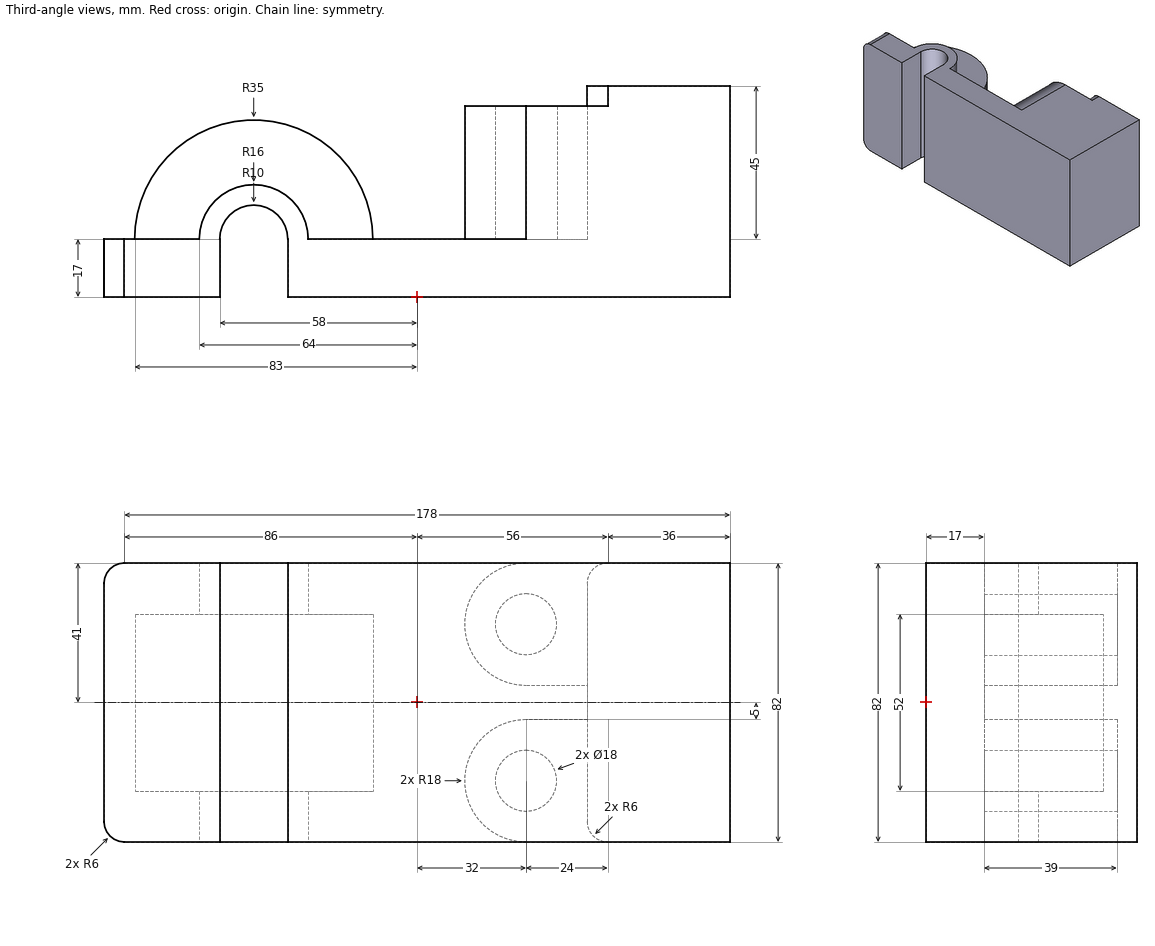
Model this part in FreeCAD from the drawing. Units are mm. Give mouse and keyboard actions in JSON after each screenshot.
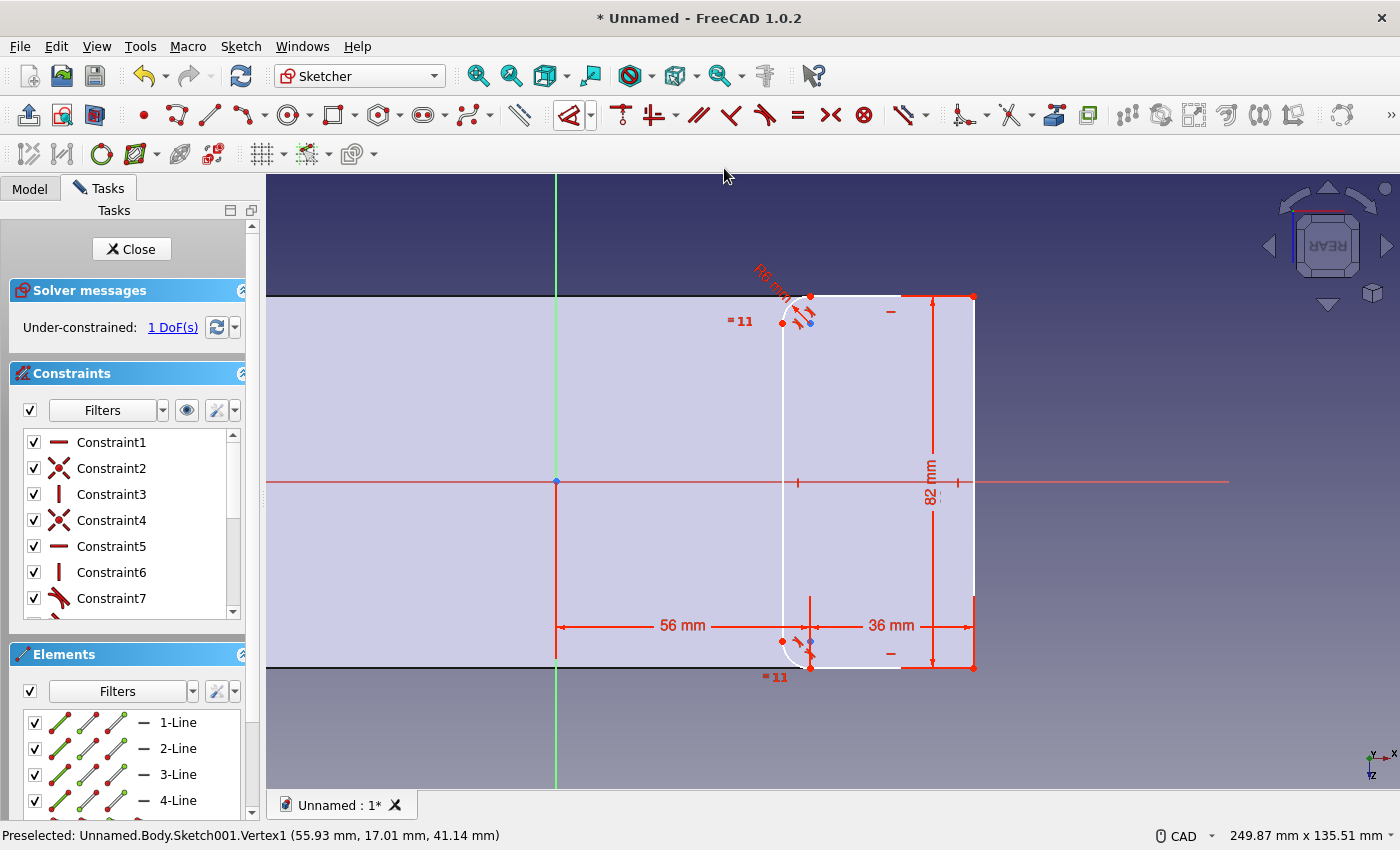
{"action": "left_click", "coordinate": [810, 668]}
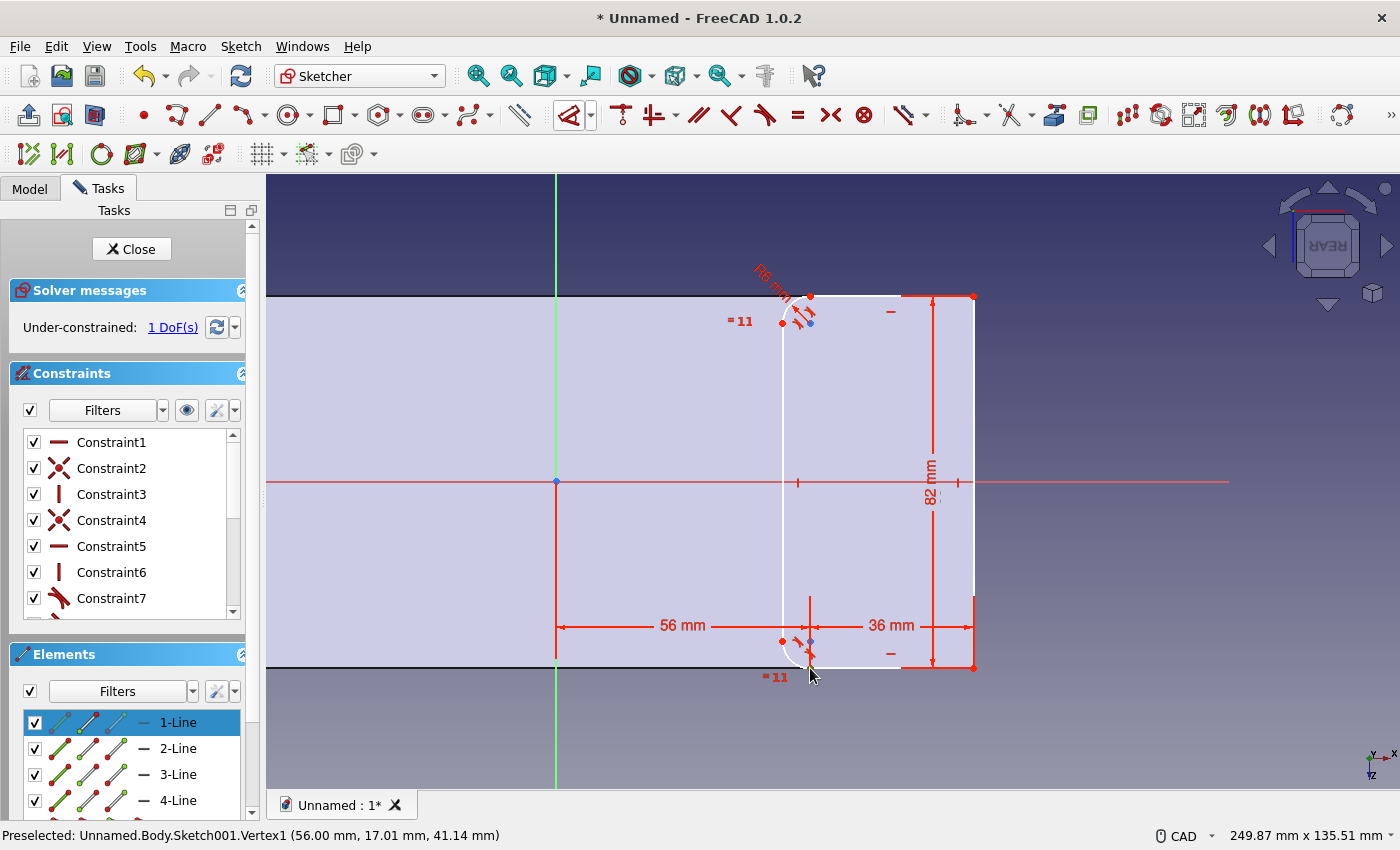
{"action": "key", "text": "i"}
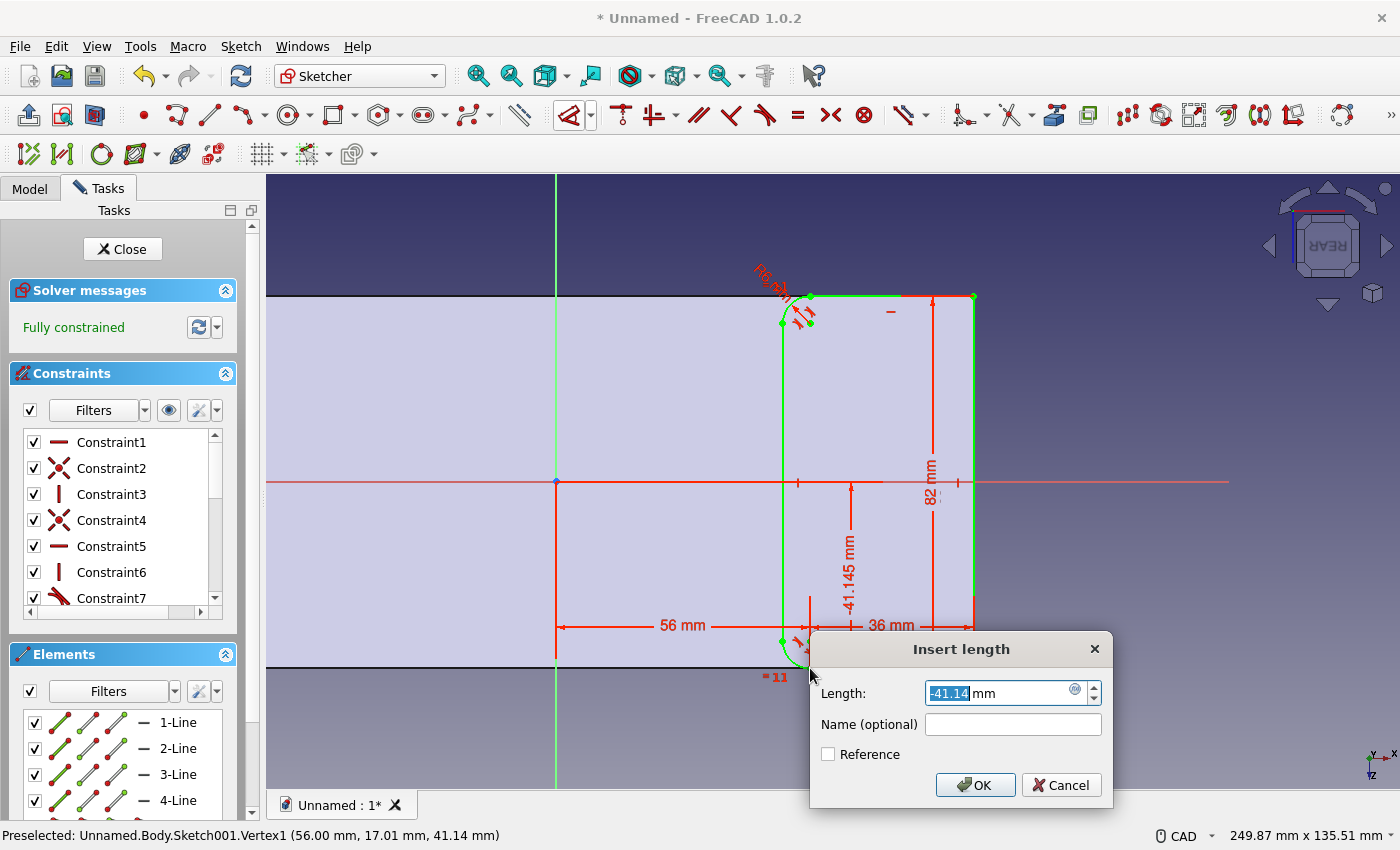
{"action": "type", "text": "-41"}
{"action": "key", "text": "Return"}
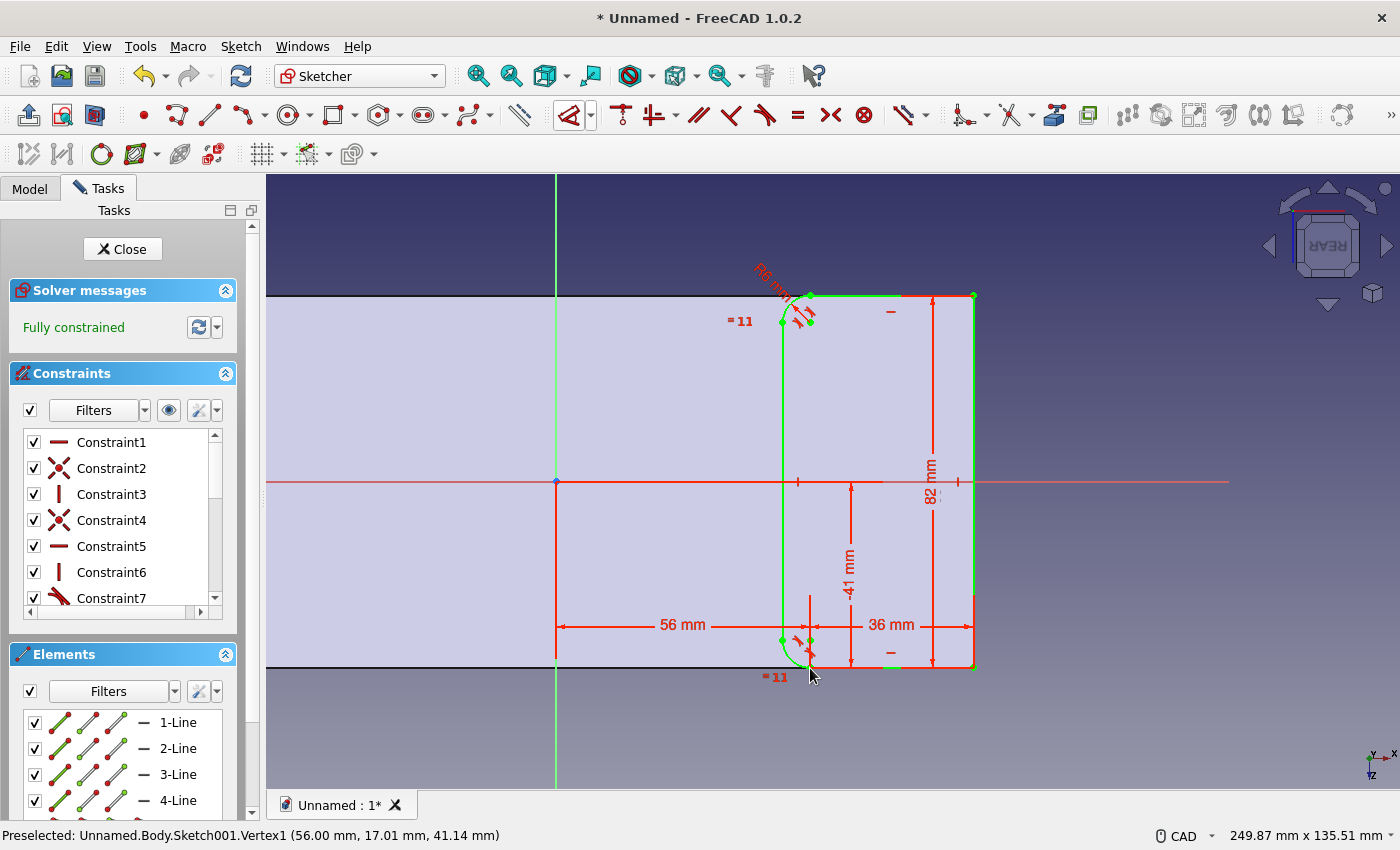
{"action": "left_click", "coordinate": [123, 249]}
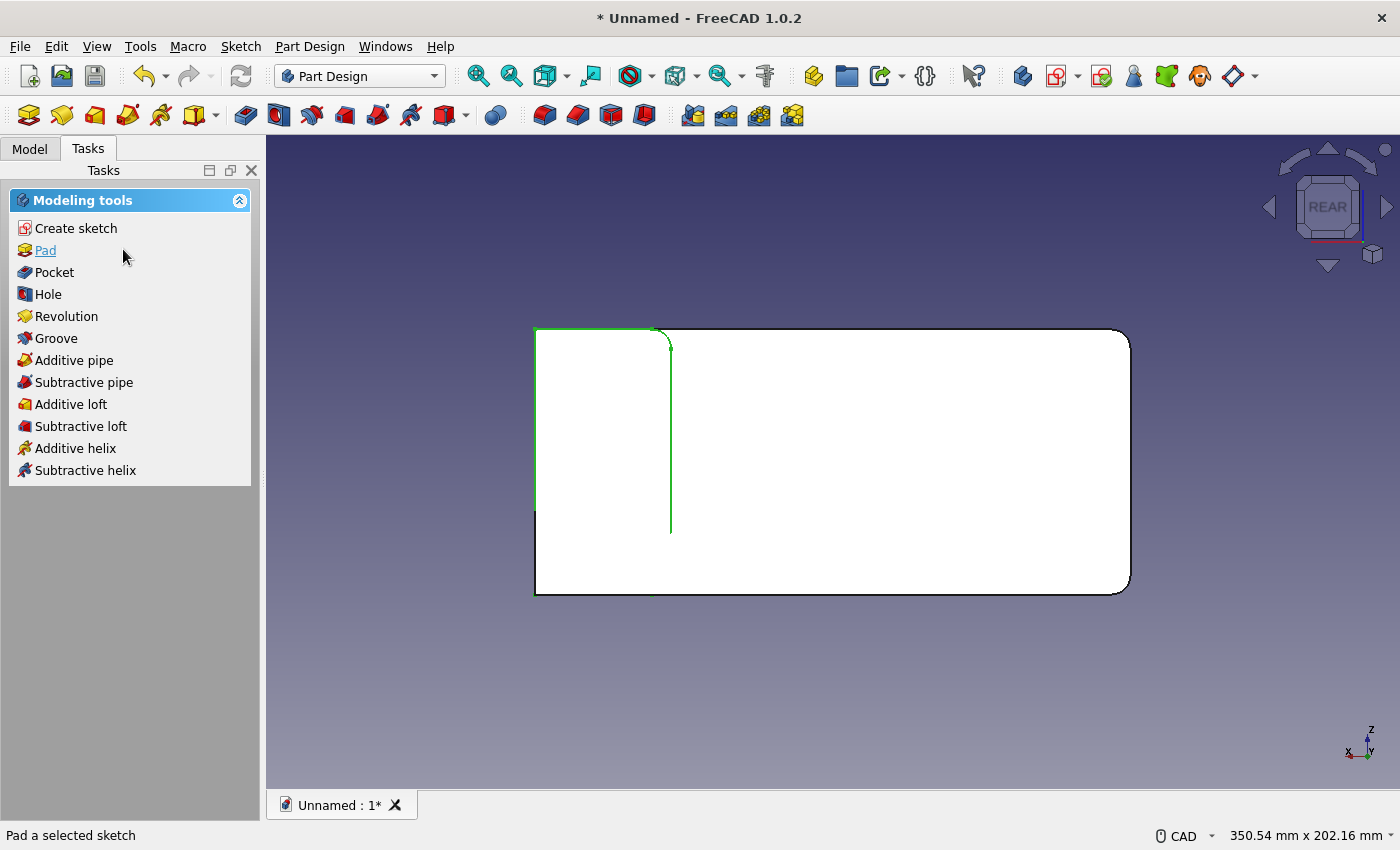
{"action": "left_click", "coordinate": [29, 116]}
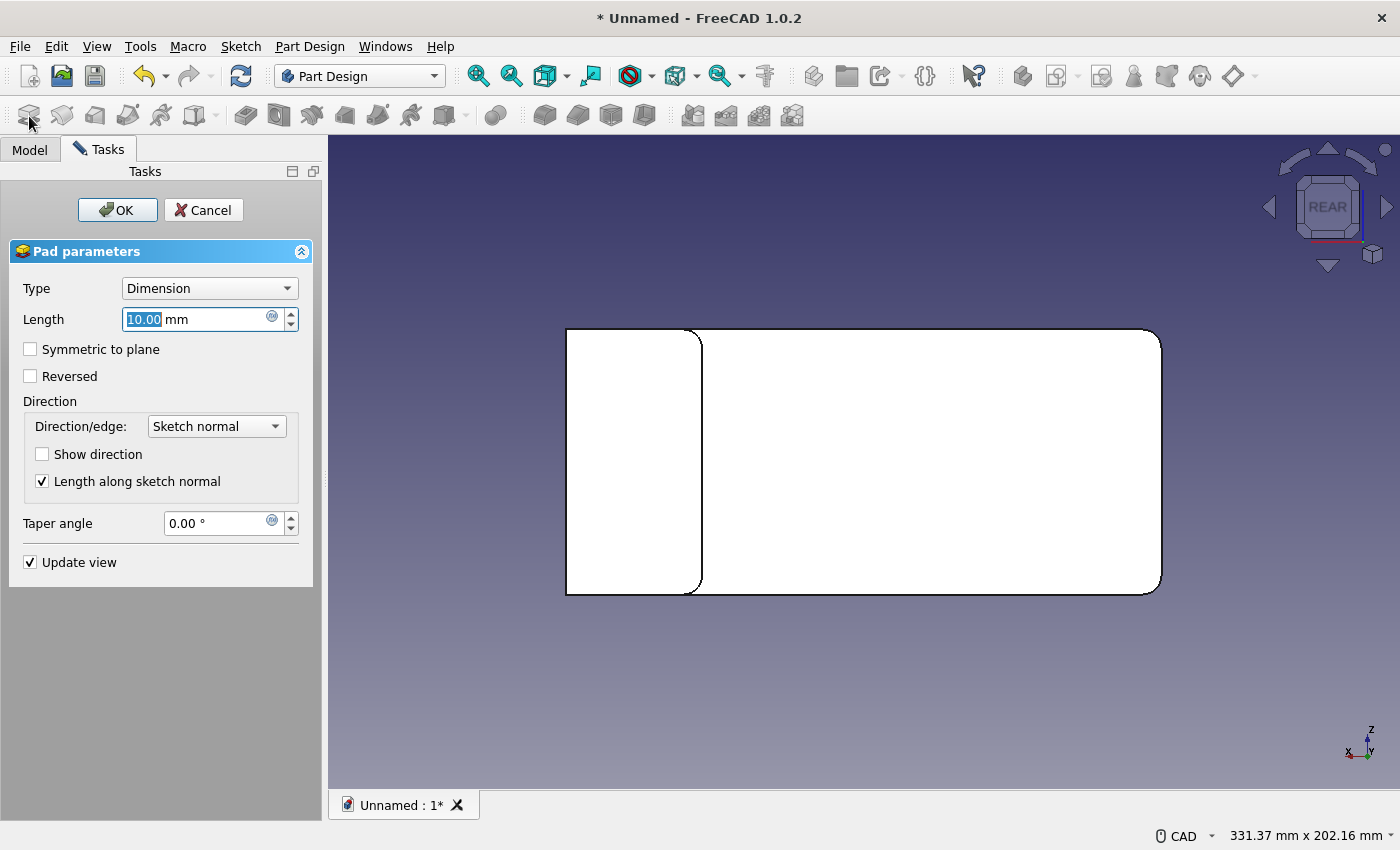
{"action": "type", "text": "45"}
{"action": "key", "text": "Tab"}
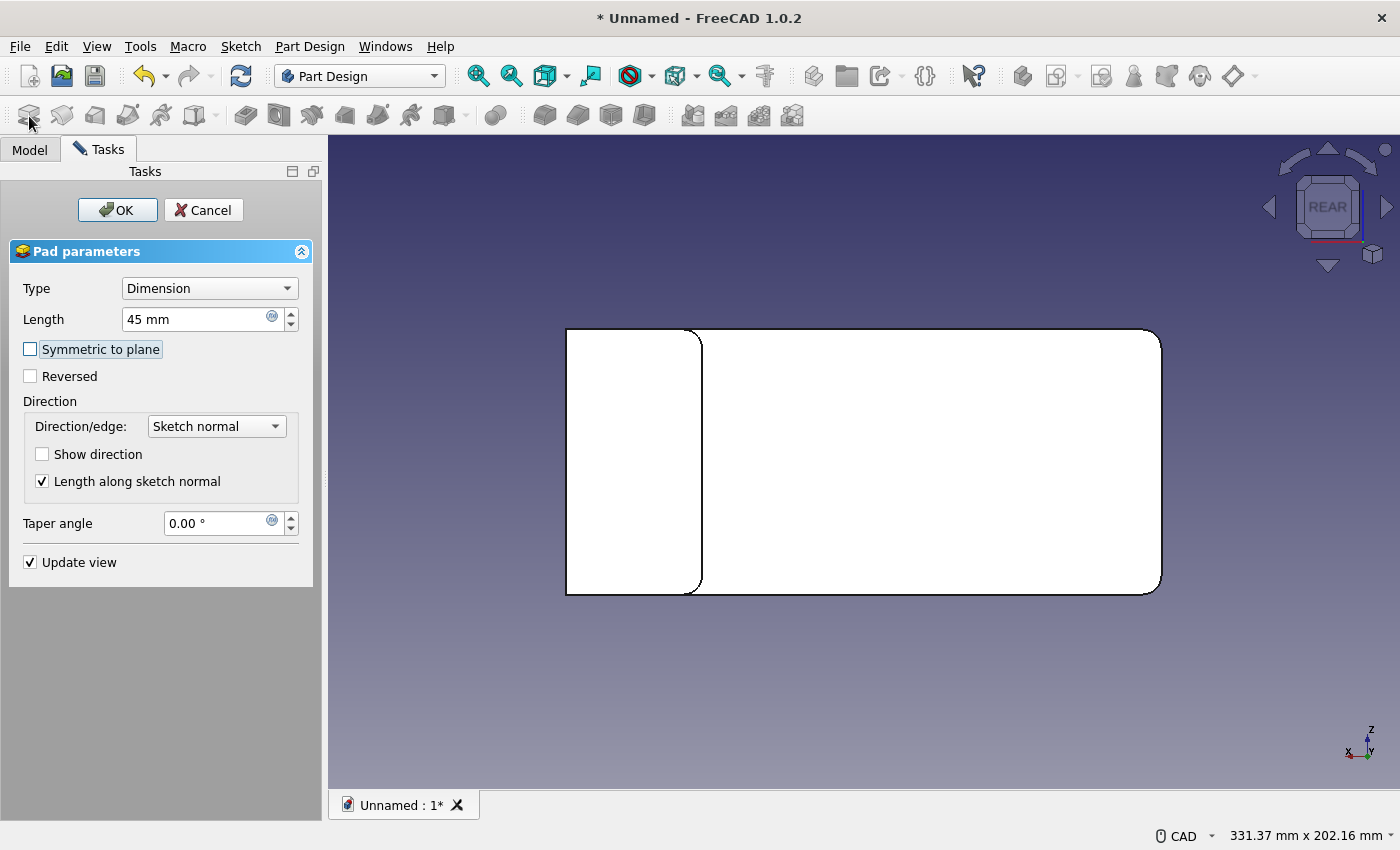
{"action": "left_click", "coordinate": [118, 210]}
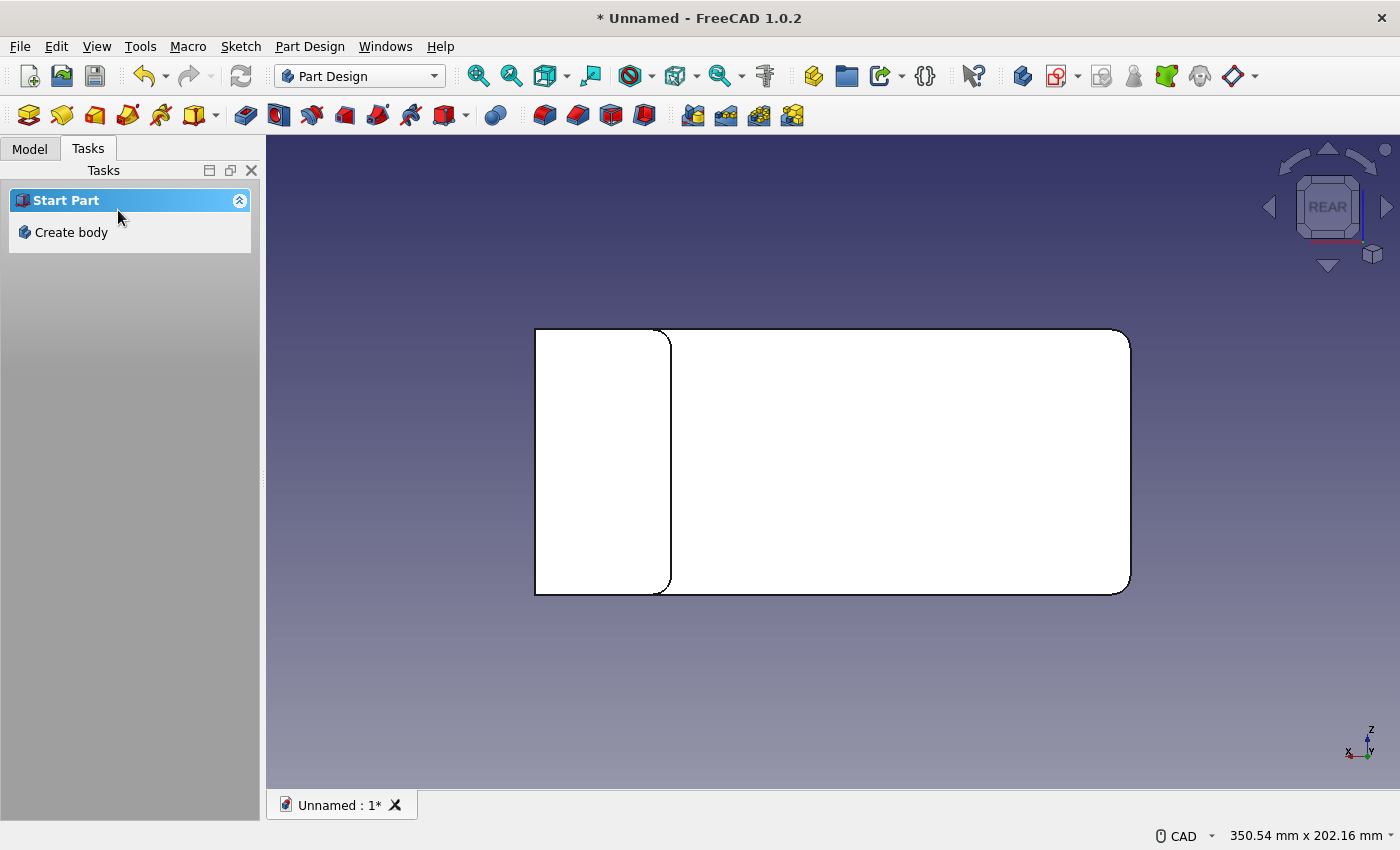
{"action": "key", "text": "0"}